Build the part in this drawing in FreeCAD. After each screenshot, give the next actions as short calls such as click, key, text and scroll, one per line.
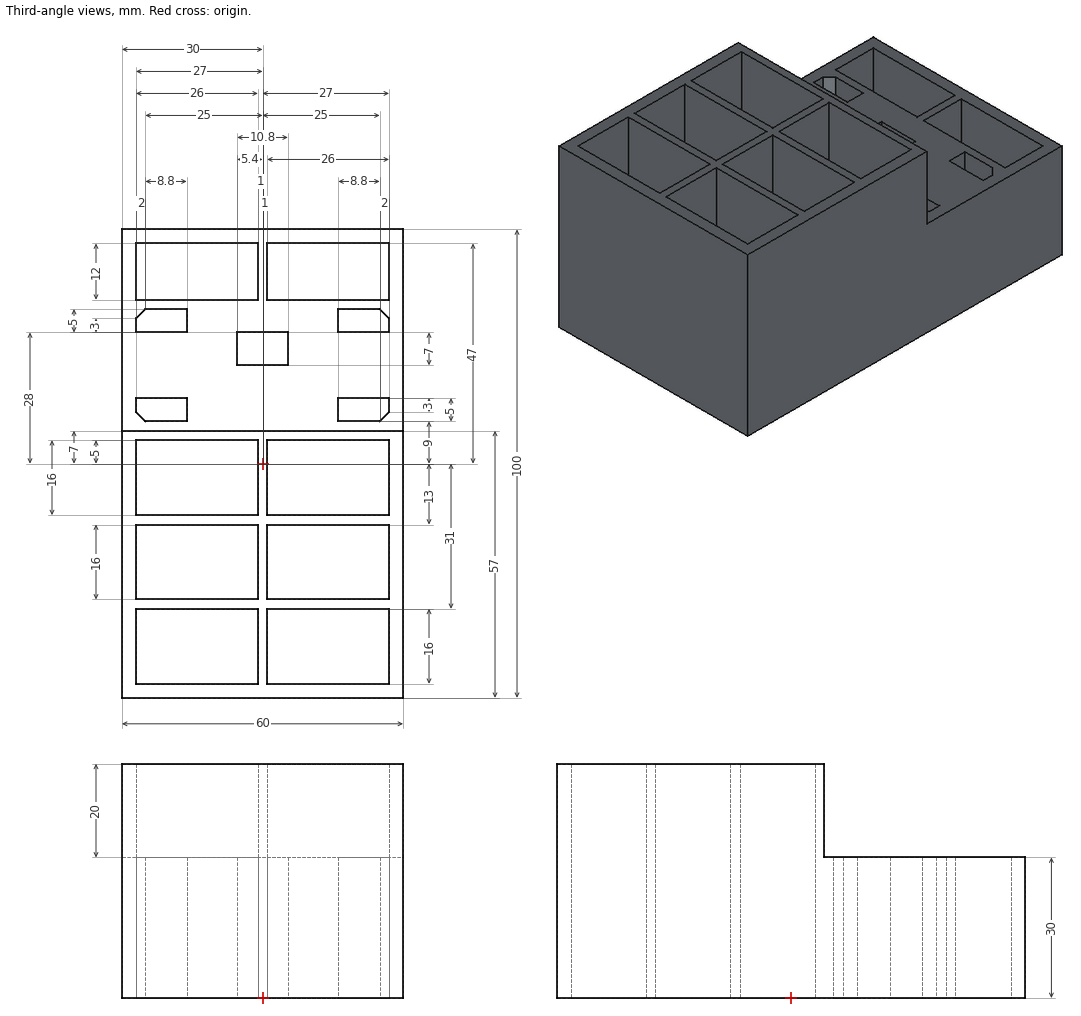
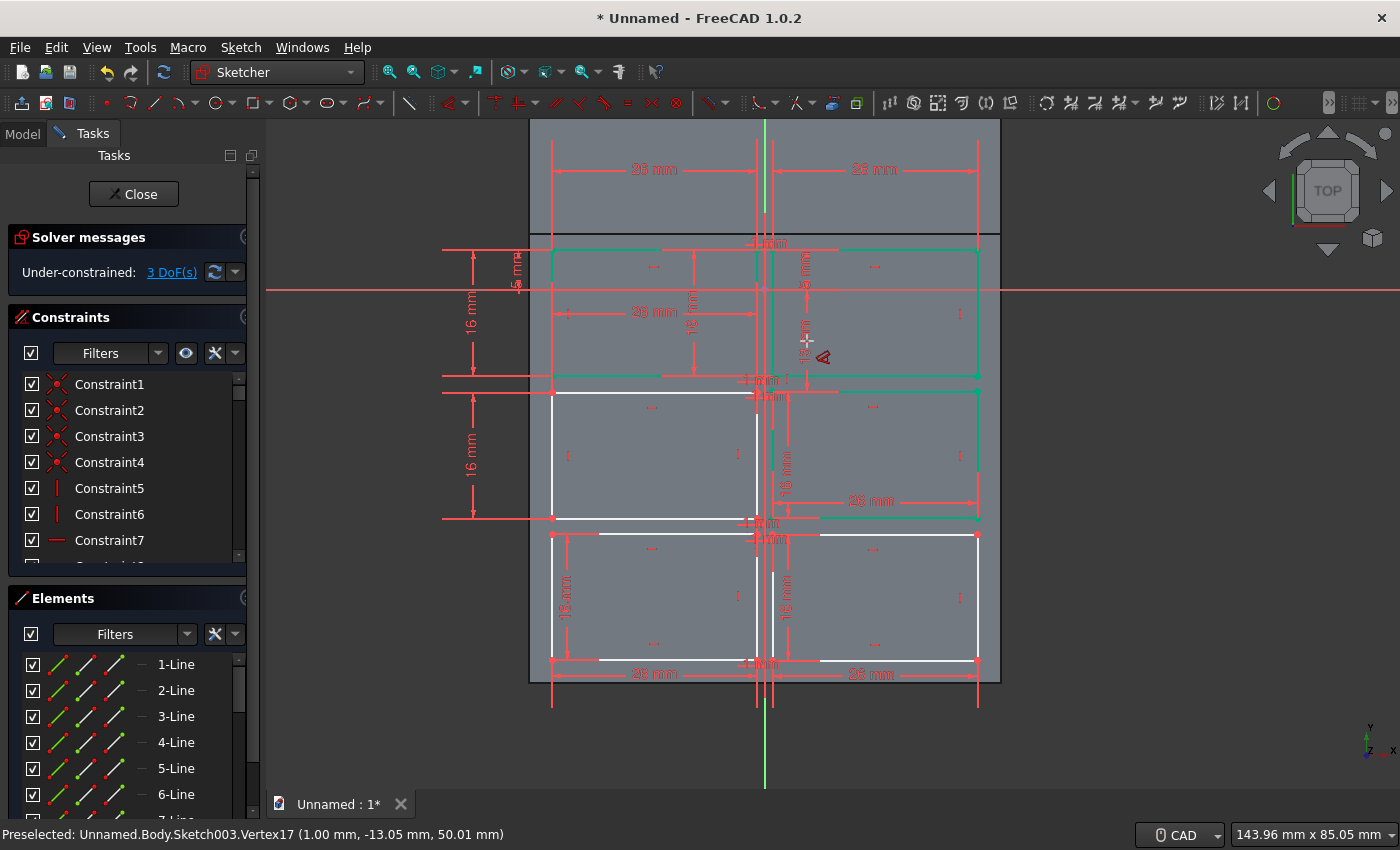
click(773, 535)
click(731, 356)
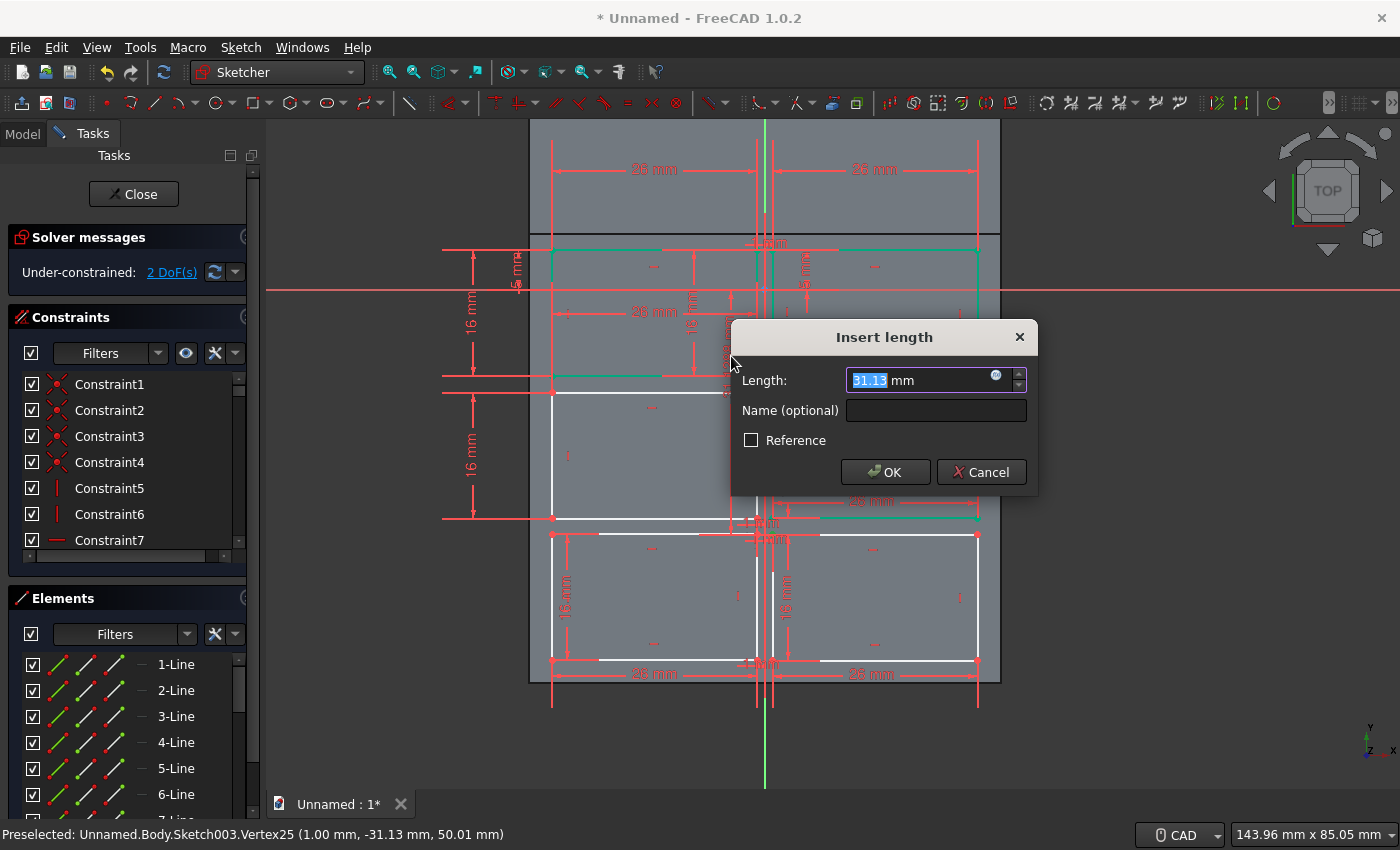
text(31)
key(Return)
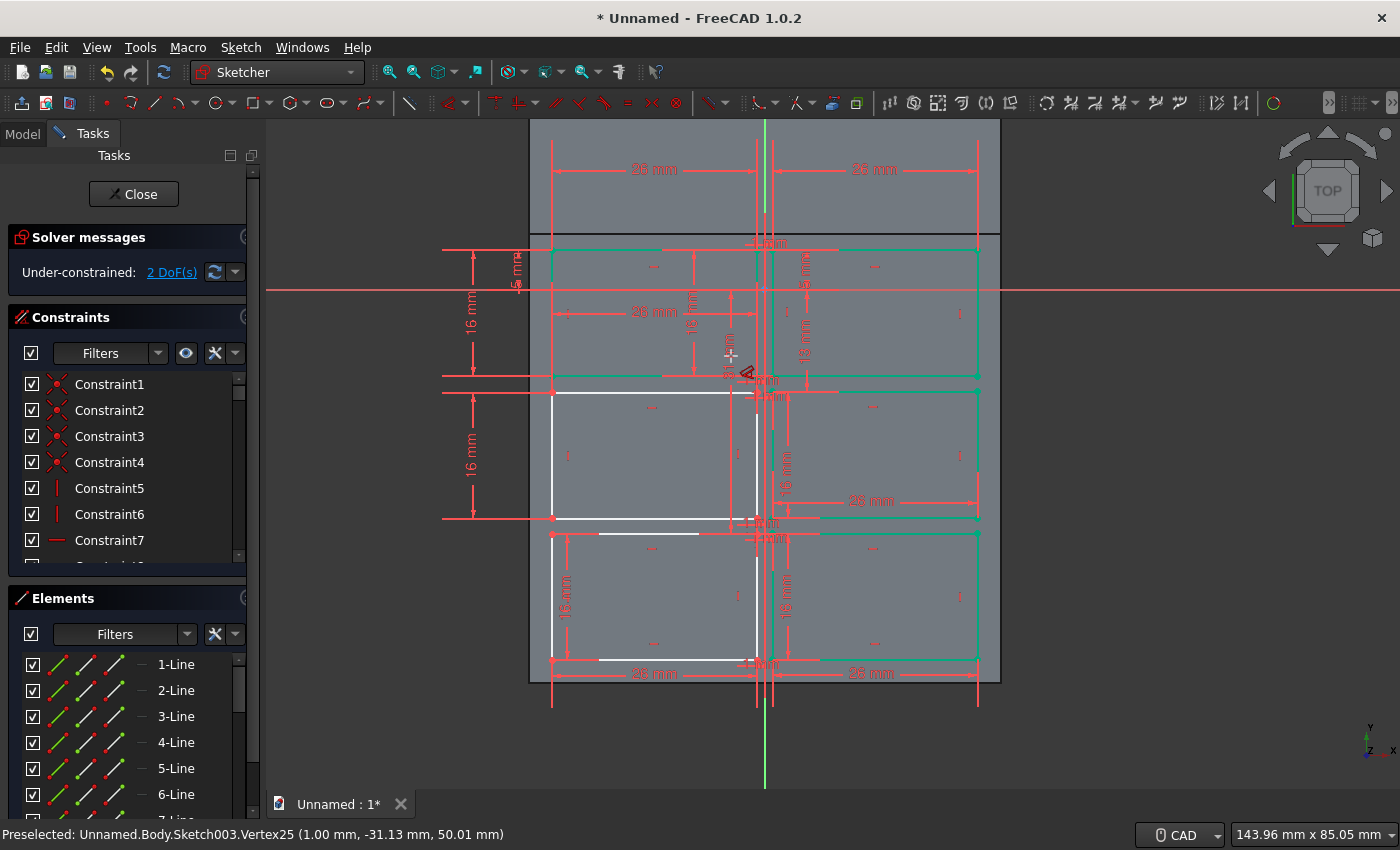
click(552, 393)
click(518, 341)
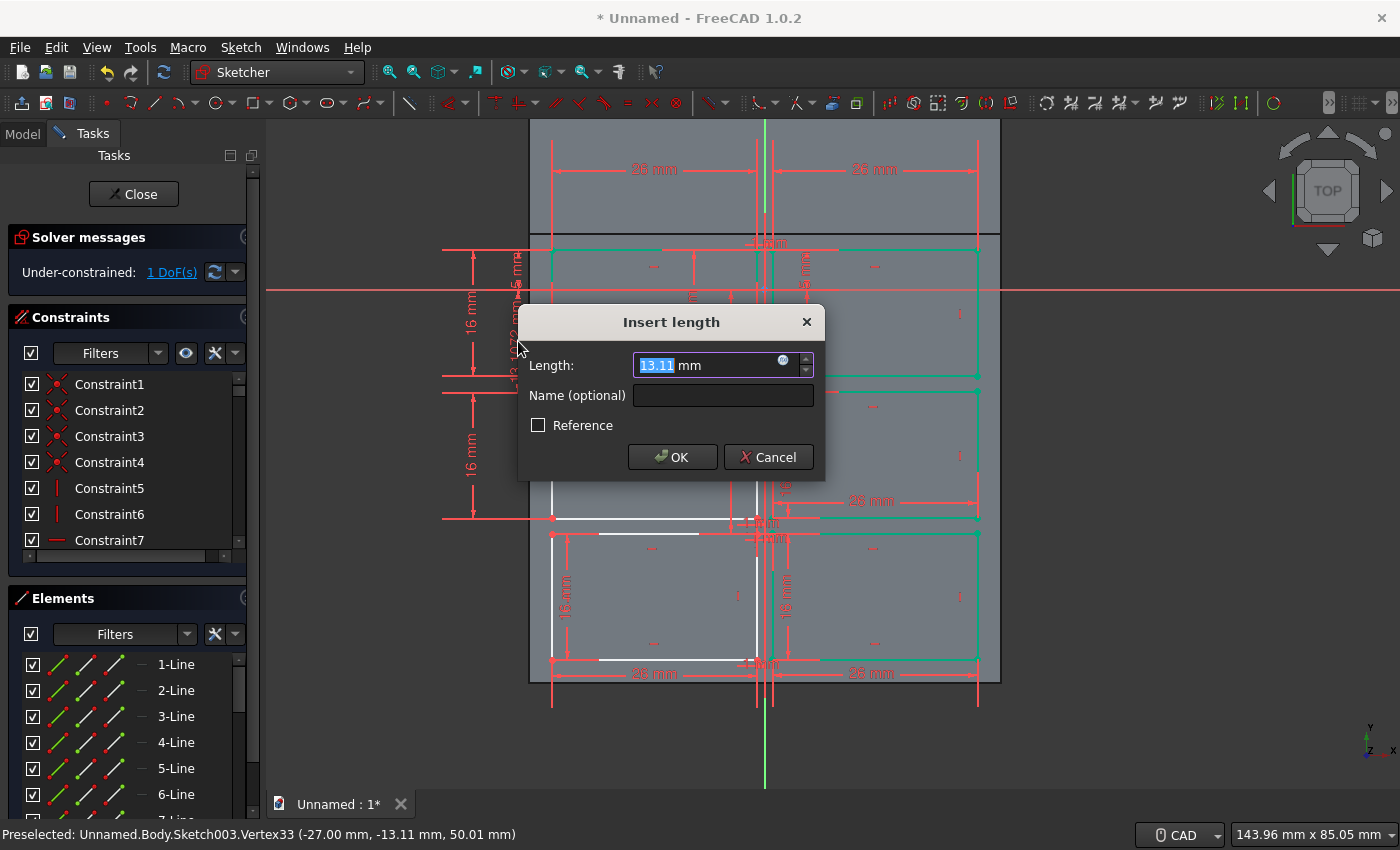
text(13)
key(Return)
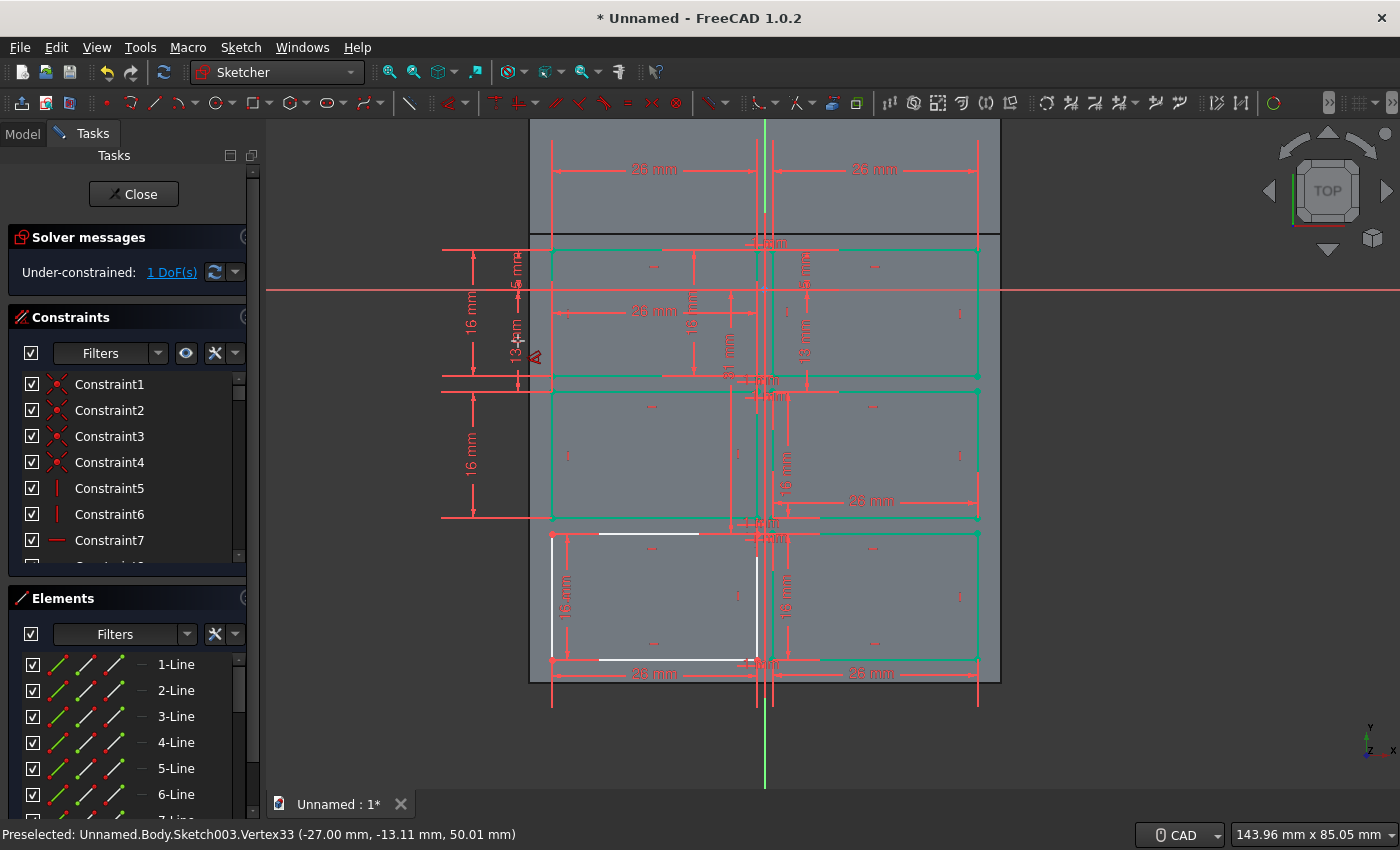
click(552, 534)
click(518, 412)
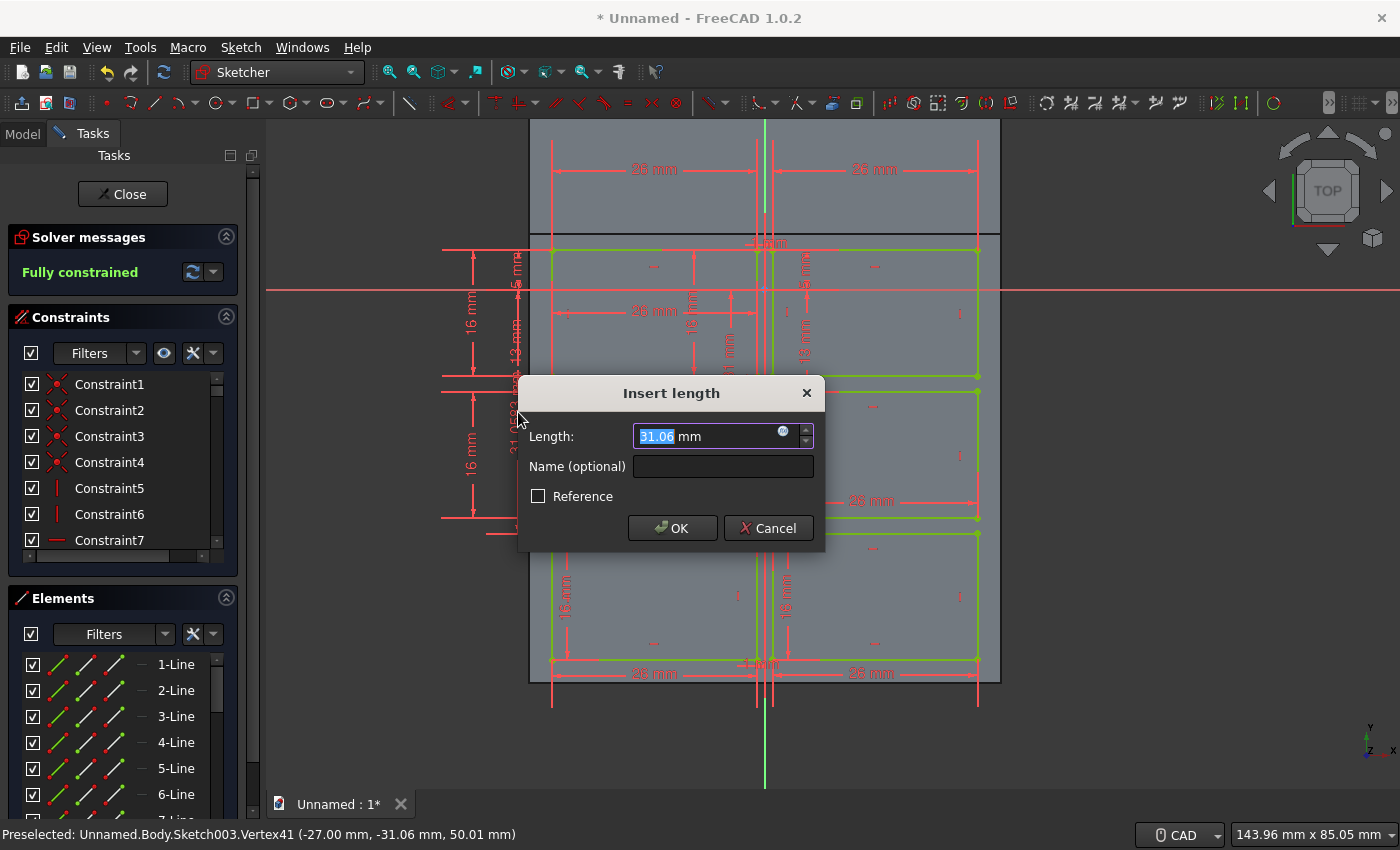
text(31)
key(Return)
key(Escape)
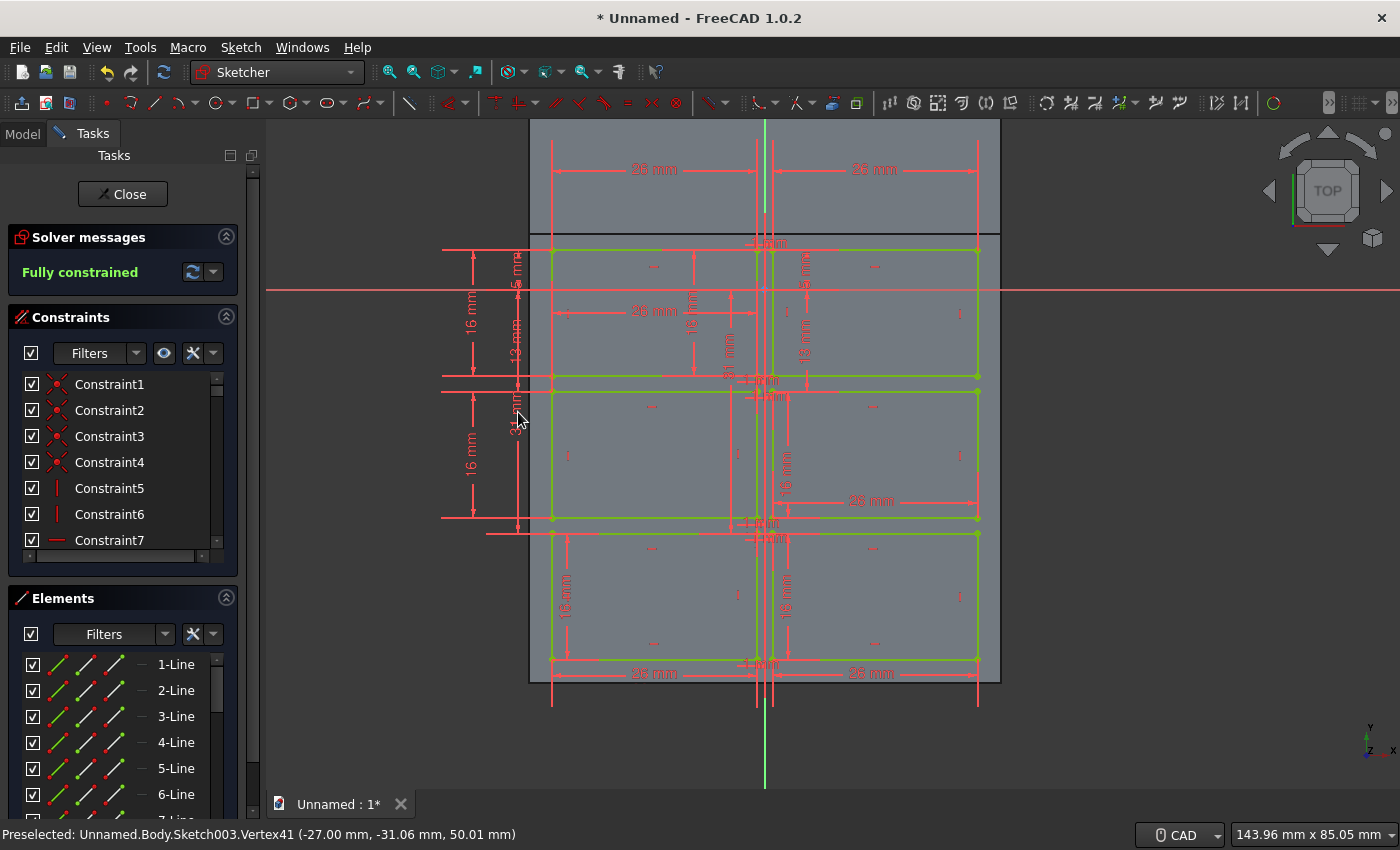
click(123, 194)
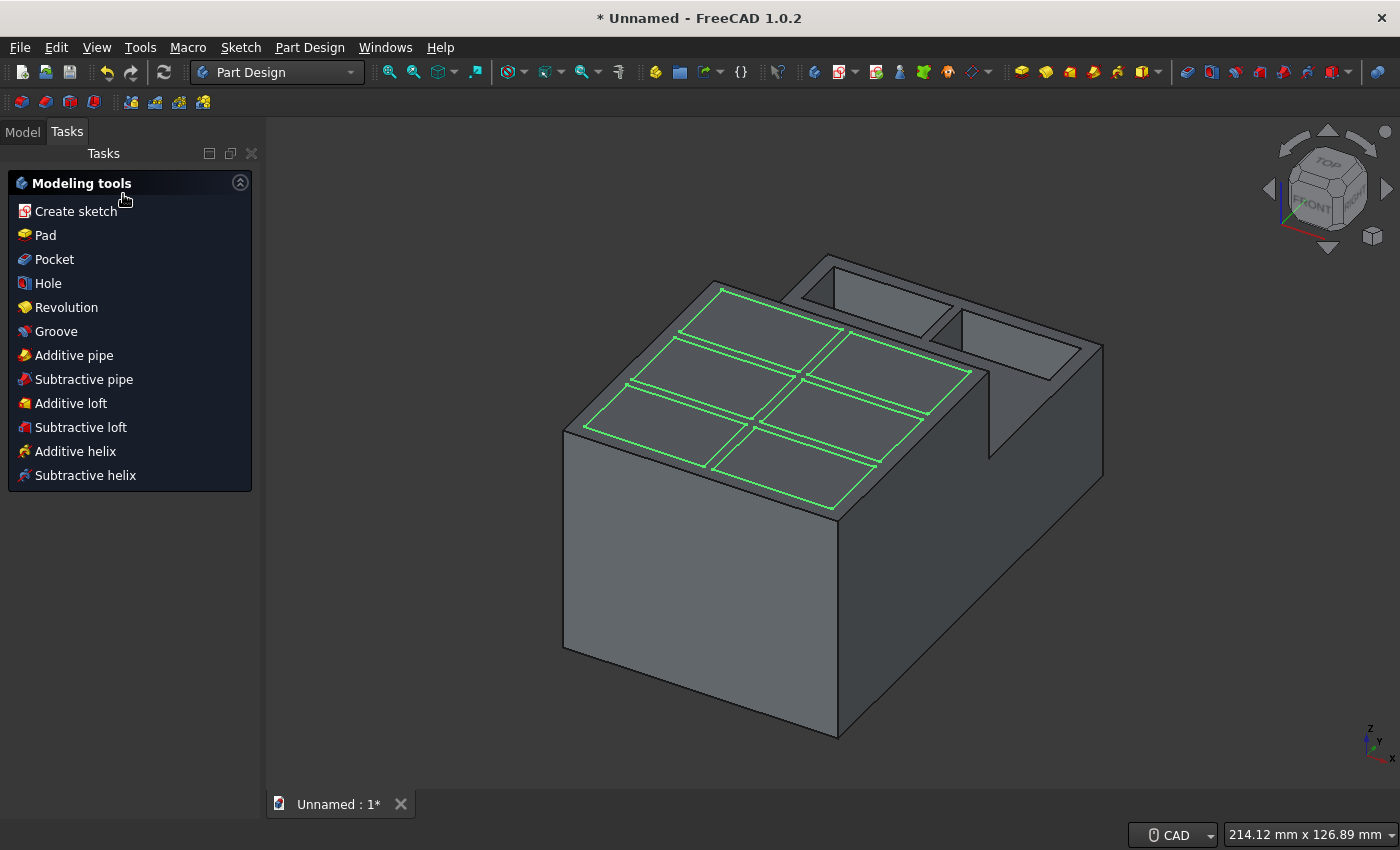
click(1188, 72)